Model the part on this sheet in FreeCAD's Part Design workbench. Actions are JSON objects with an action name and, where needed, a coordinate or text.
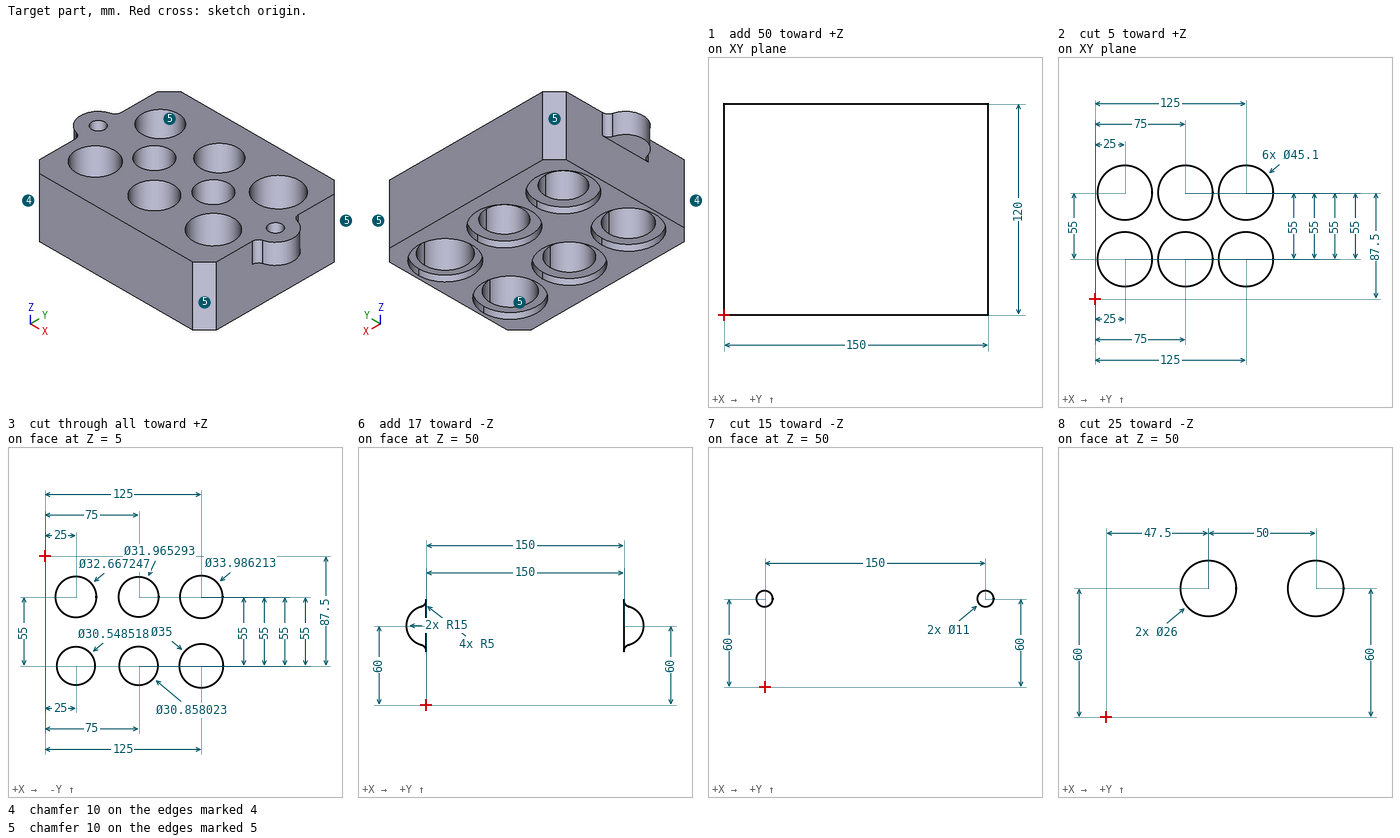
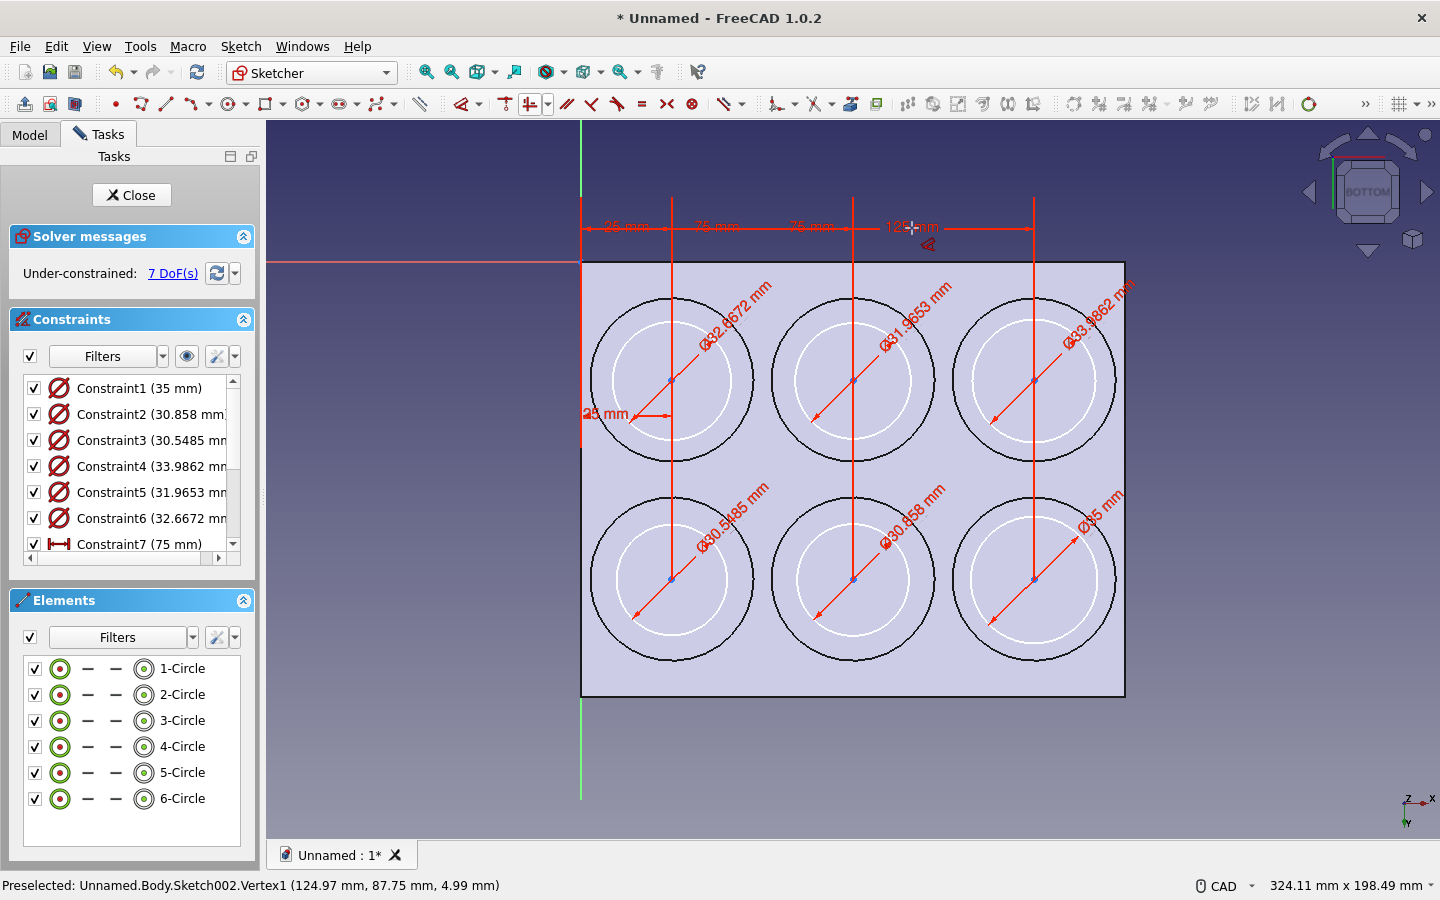
{"action": "left_click", "coordinate": [1034, 381]}
{"action": "left_click", "coordinate": [966, 415]}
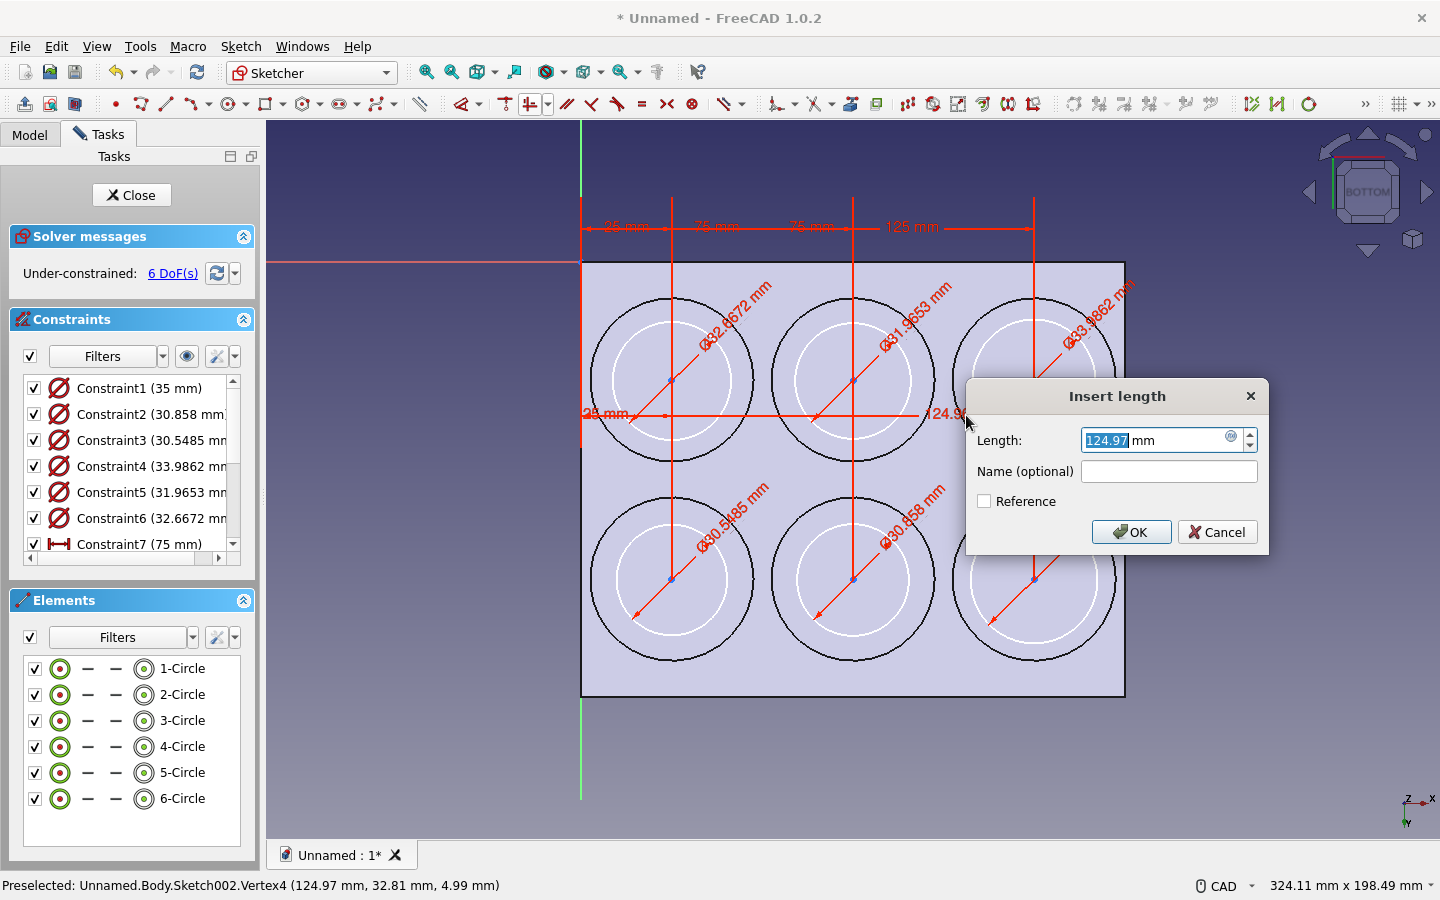
{"action": "type", "text": "125"}
{"action": "key", "text": "Return"}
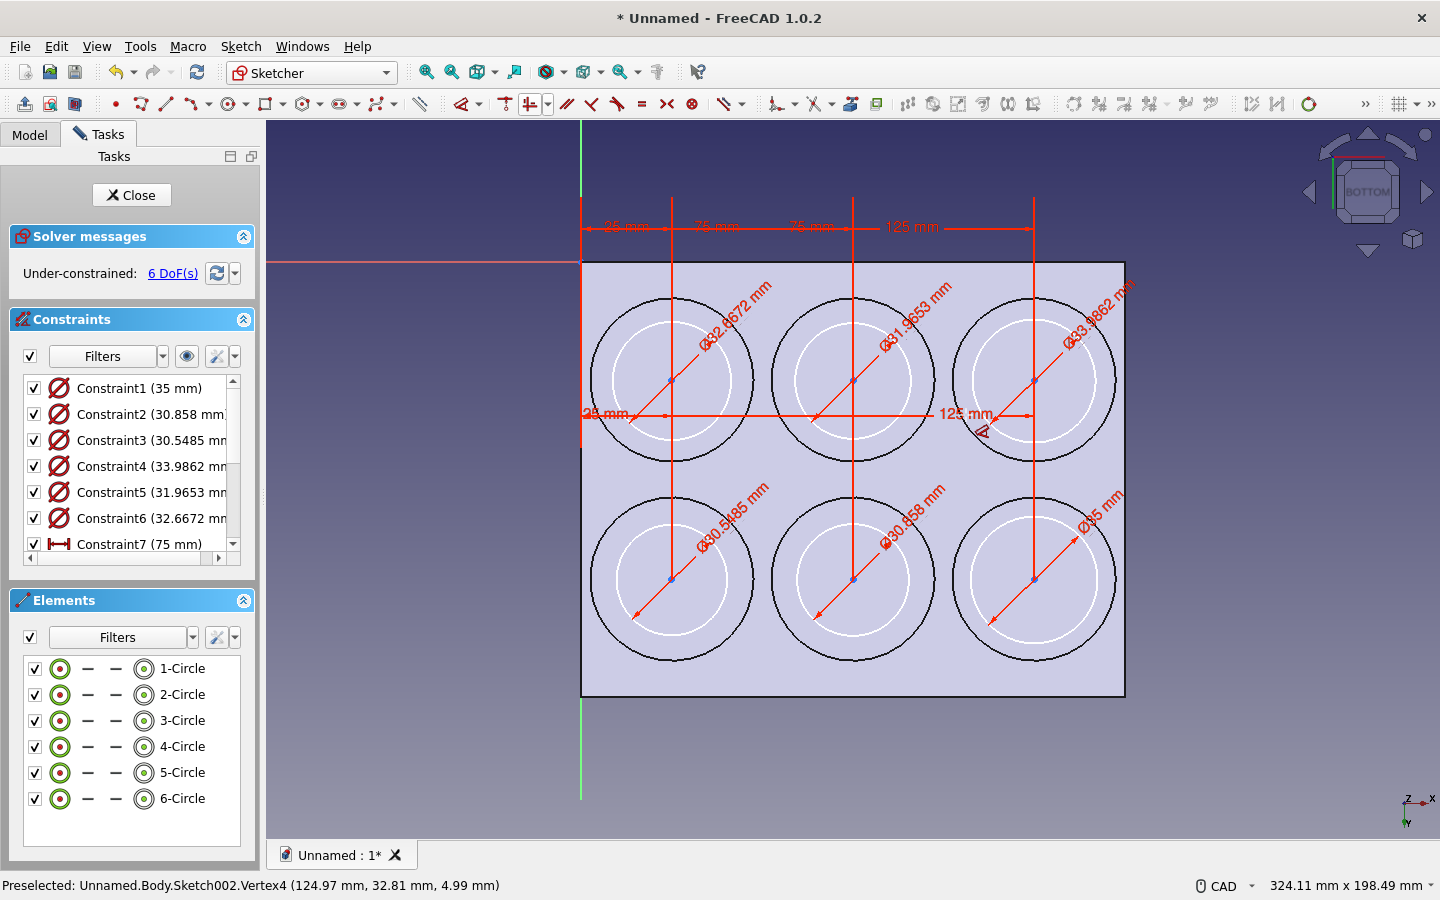
{"action": "left_click", "coordinate": [1034, 580]}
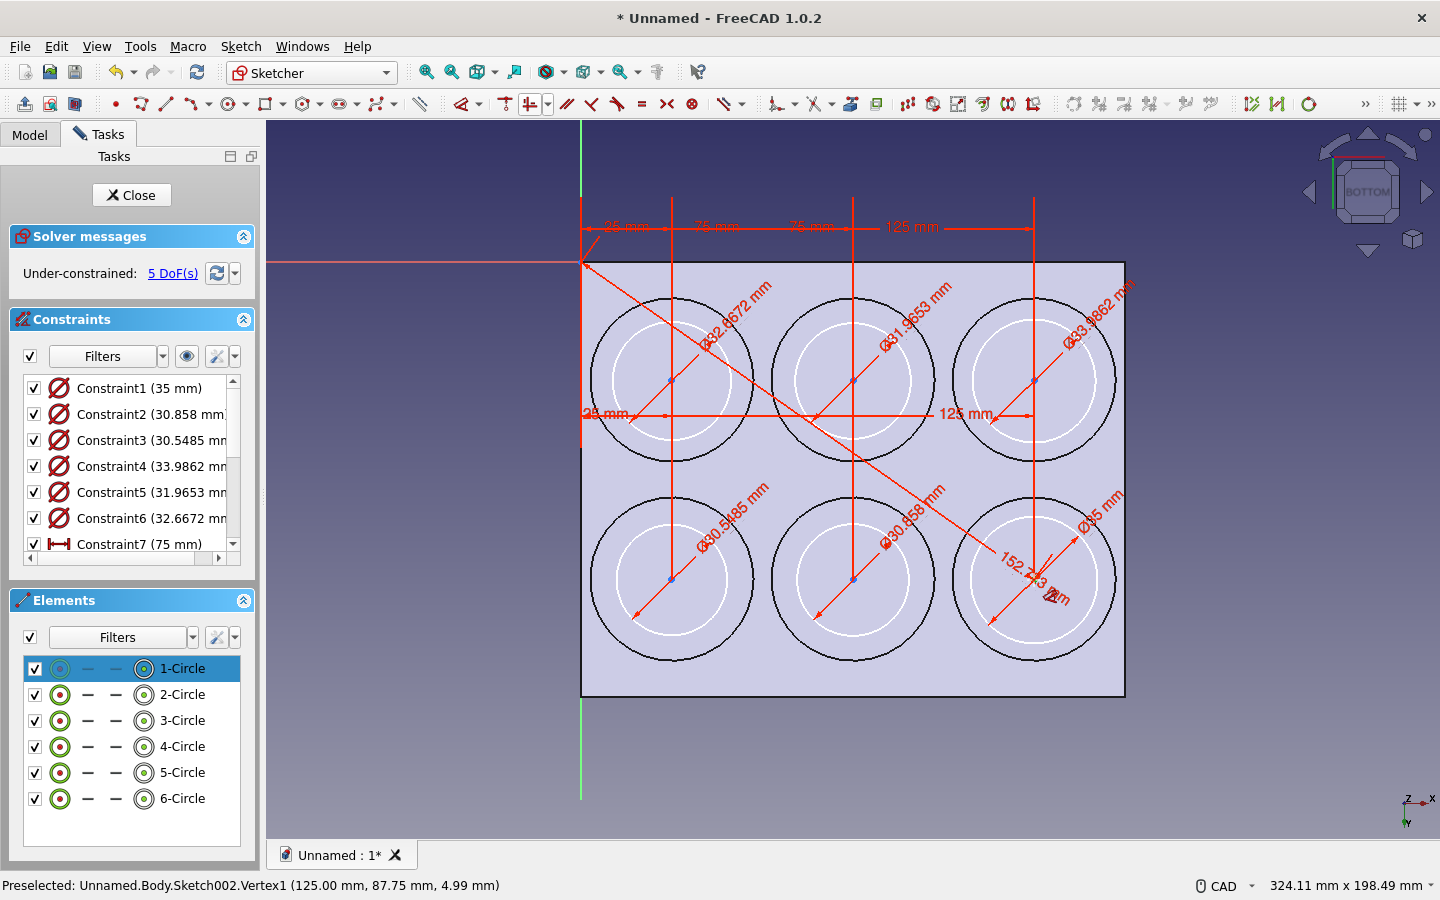
{"action": "left_click", "coordinate": [1034, 381]}
{"action": "left_click", "coordinate": [1068, 480]}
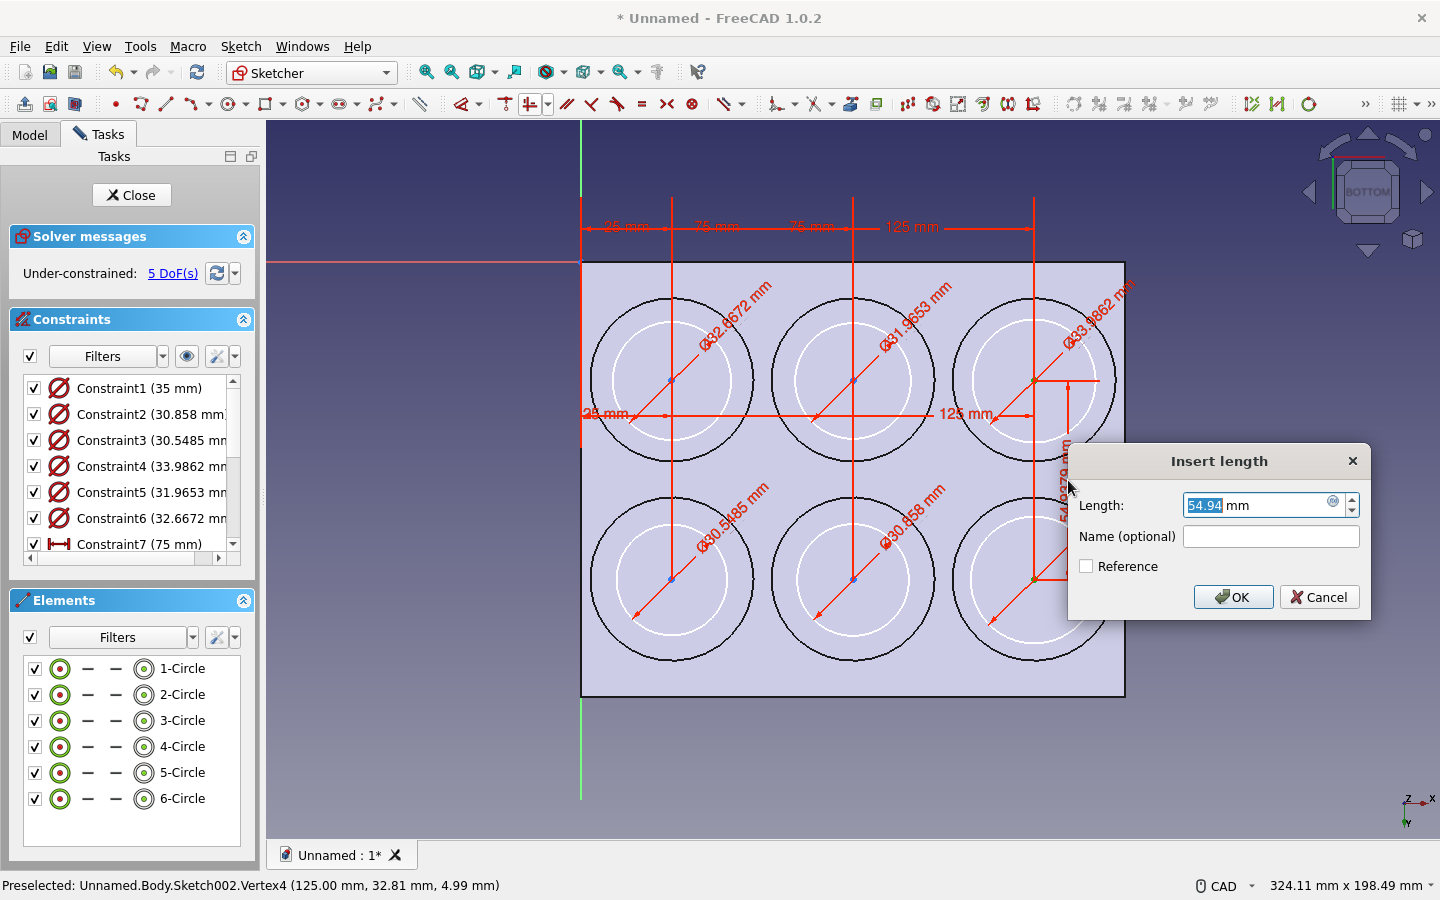
{"action": "type", "text": "55"}
{"action": "key", "text": "Return"}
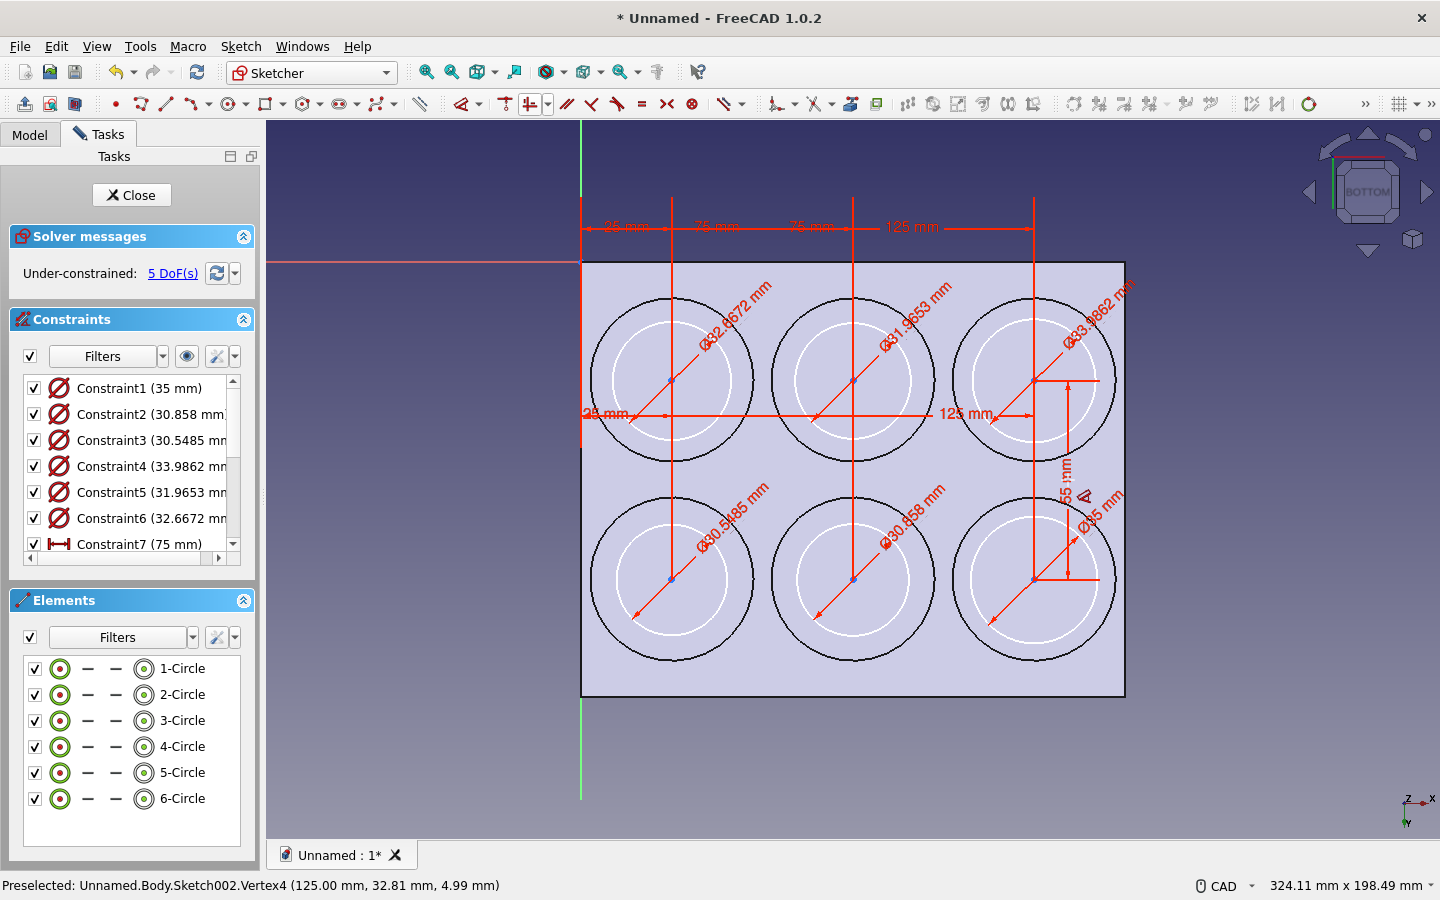
{"action": "left_click", "coordinate": [853, 580]}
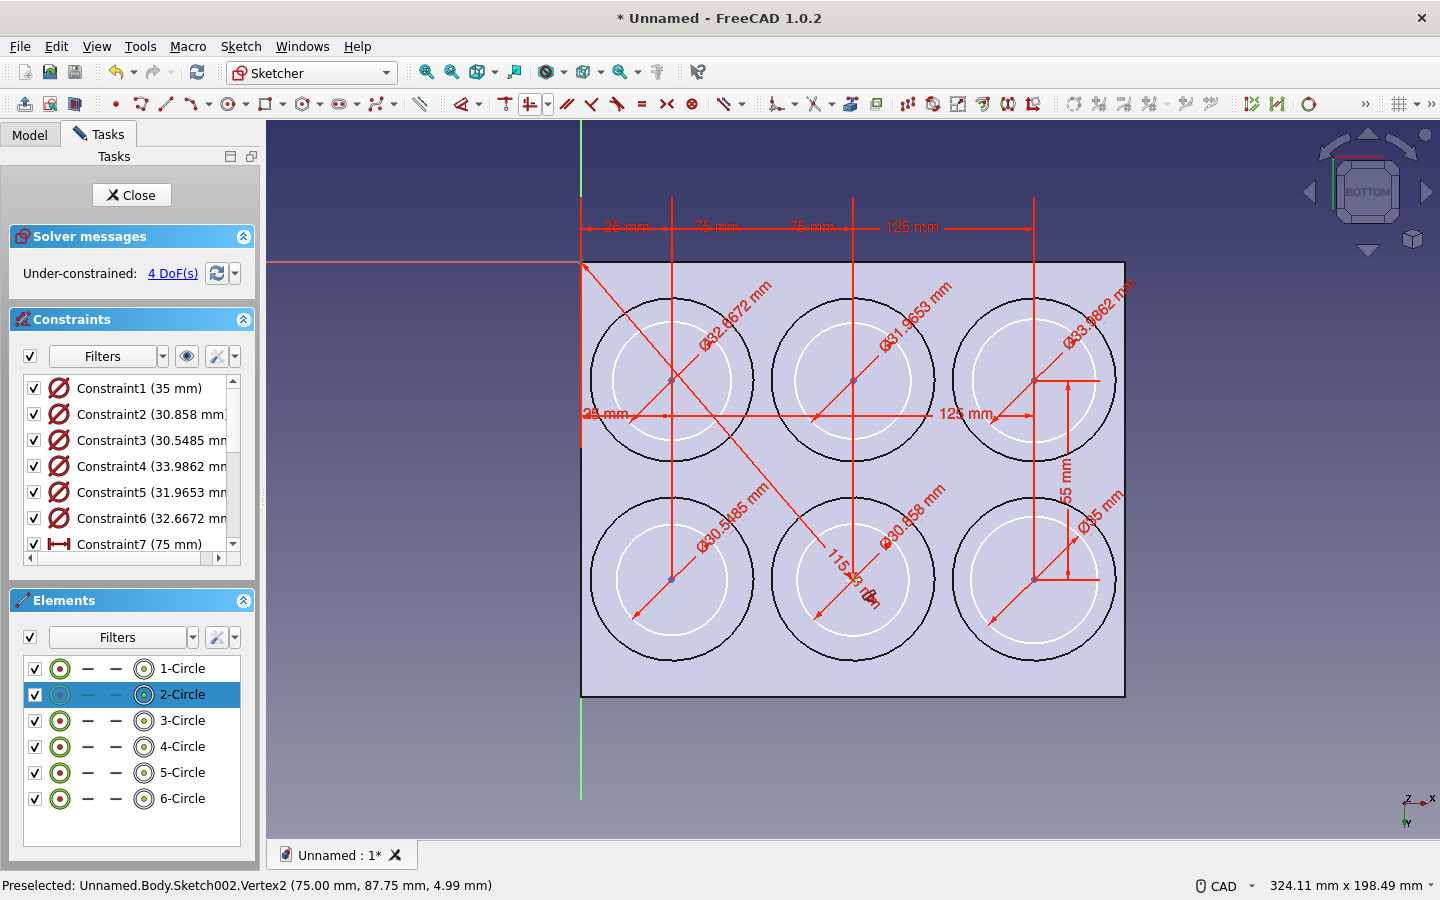
{"action": "left_click", "coordinate": [1034, 381]}
{"action": "left_click", "coordinate": [1068, 411]}